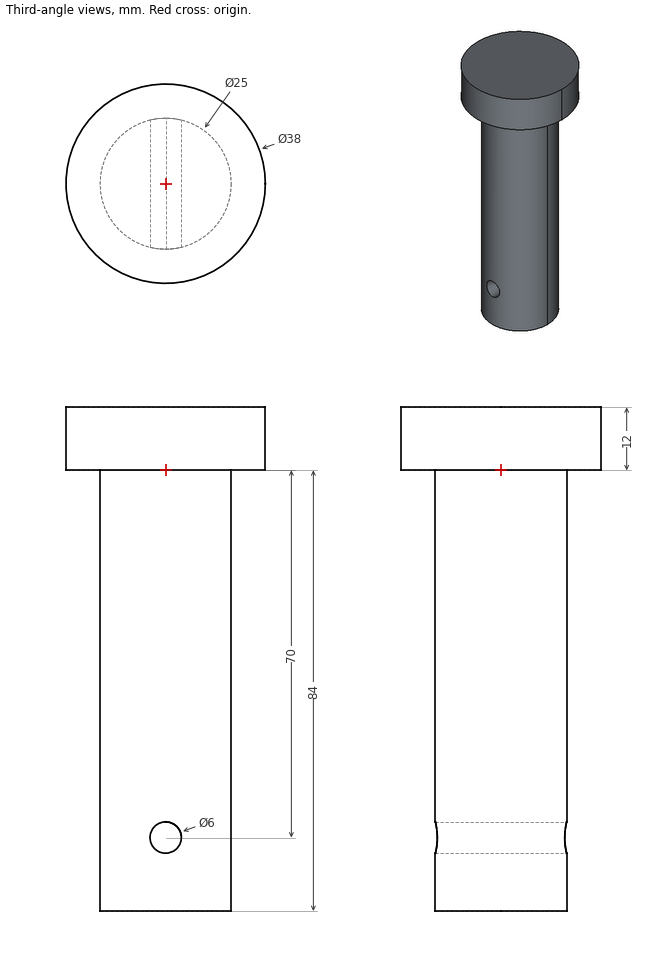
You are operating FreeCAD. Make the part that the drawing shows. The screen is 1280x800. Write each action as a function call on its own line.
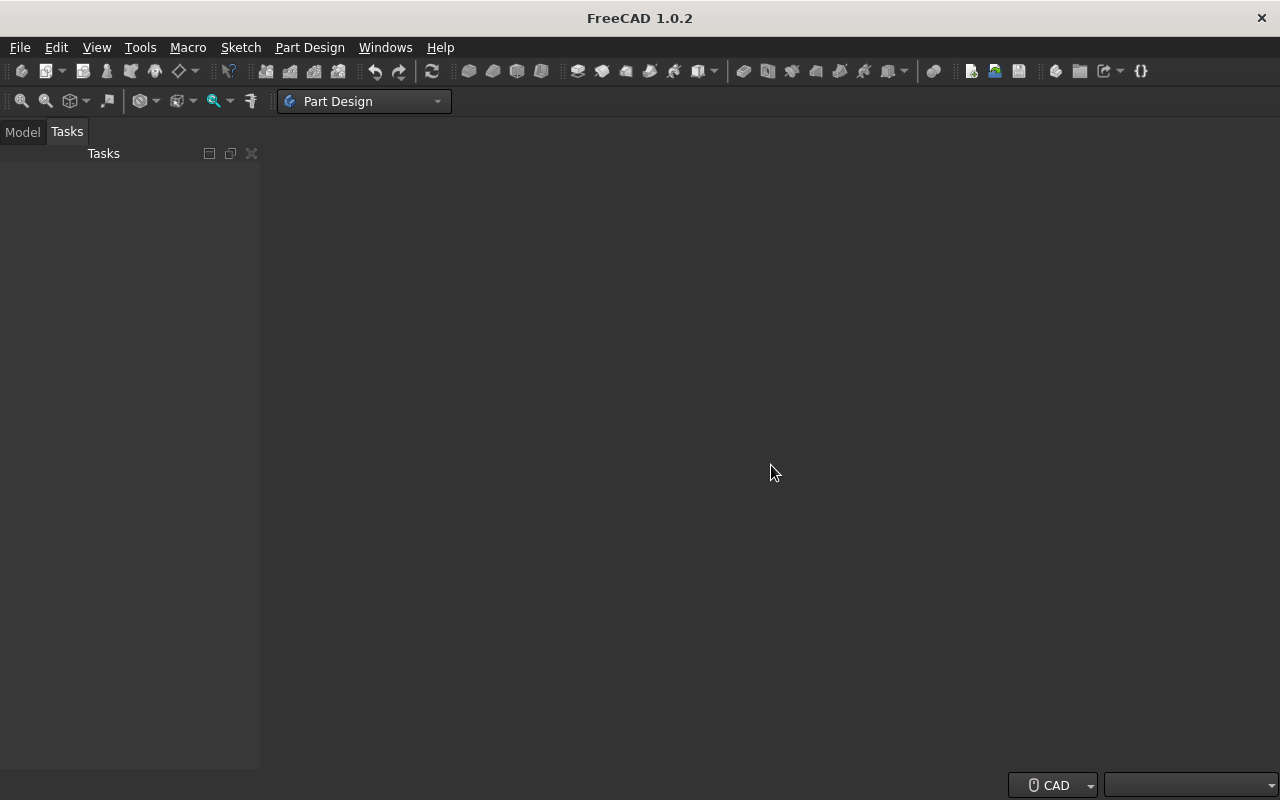
click(972, 72)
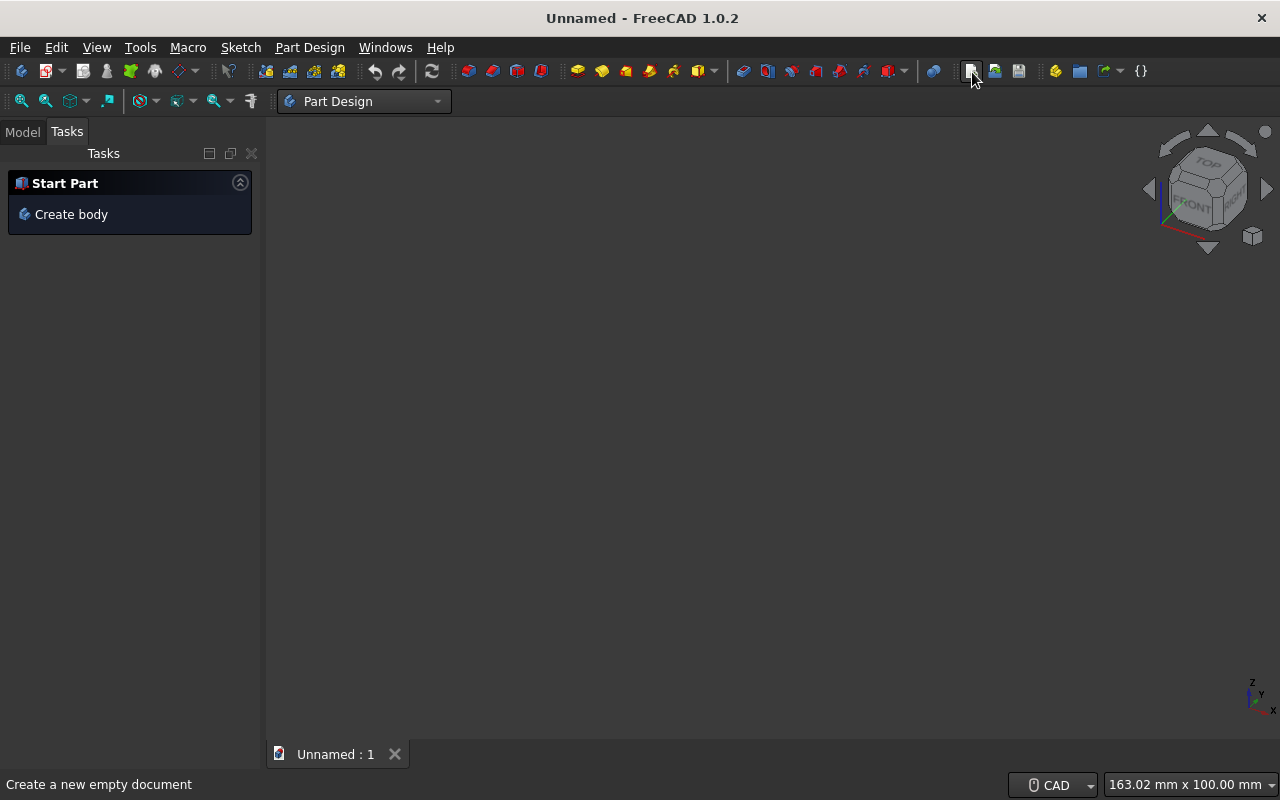
click(46, 72)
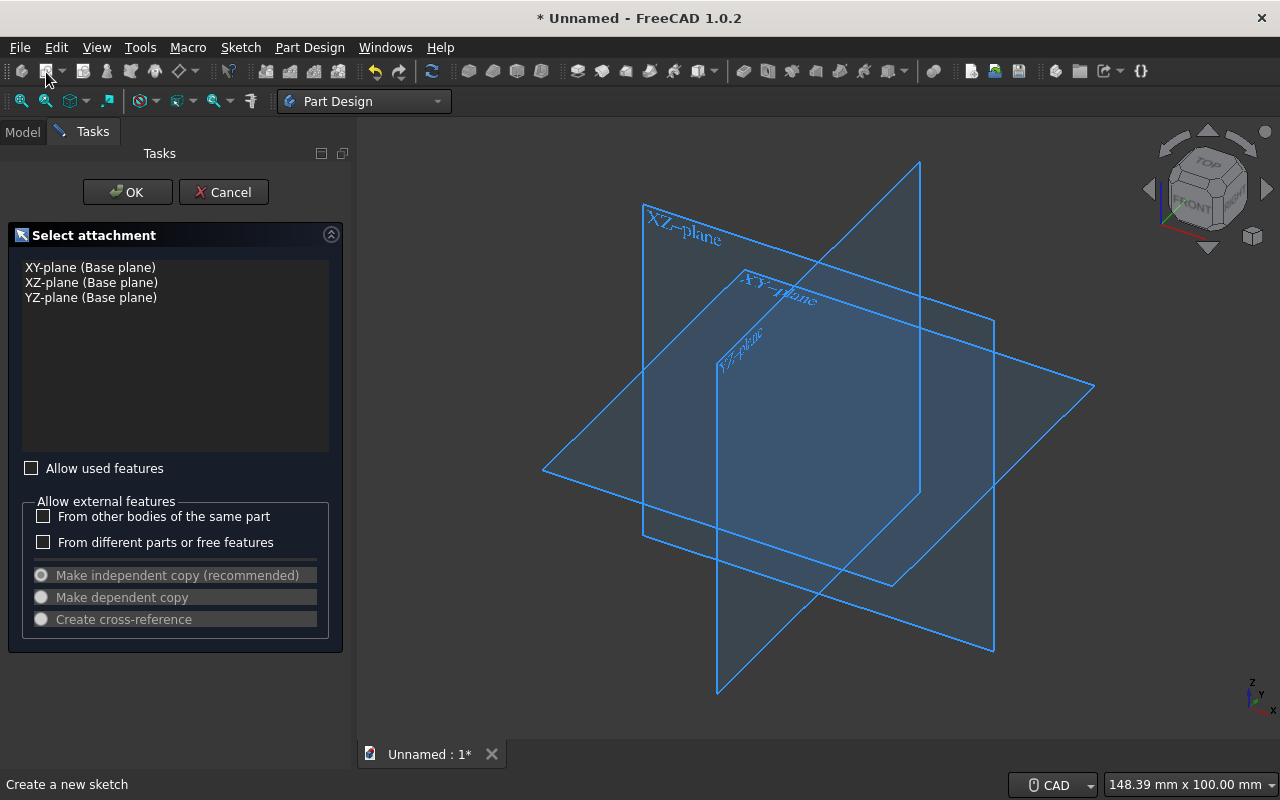
click(82, 268)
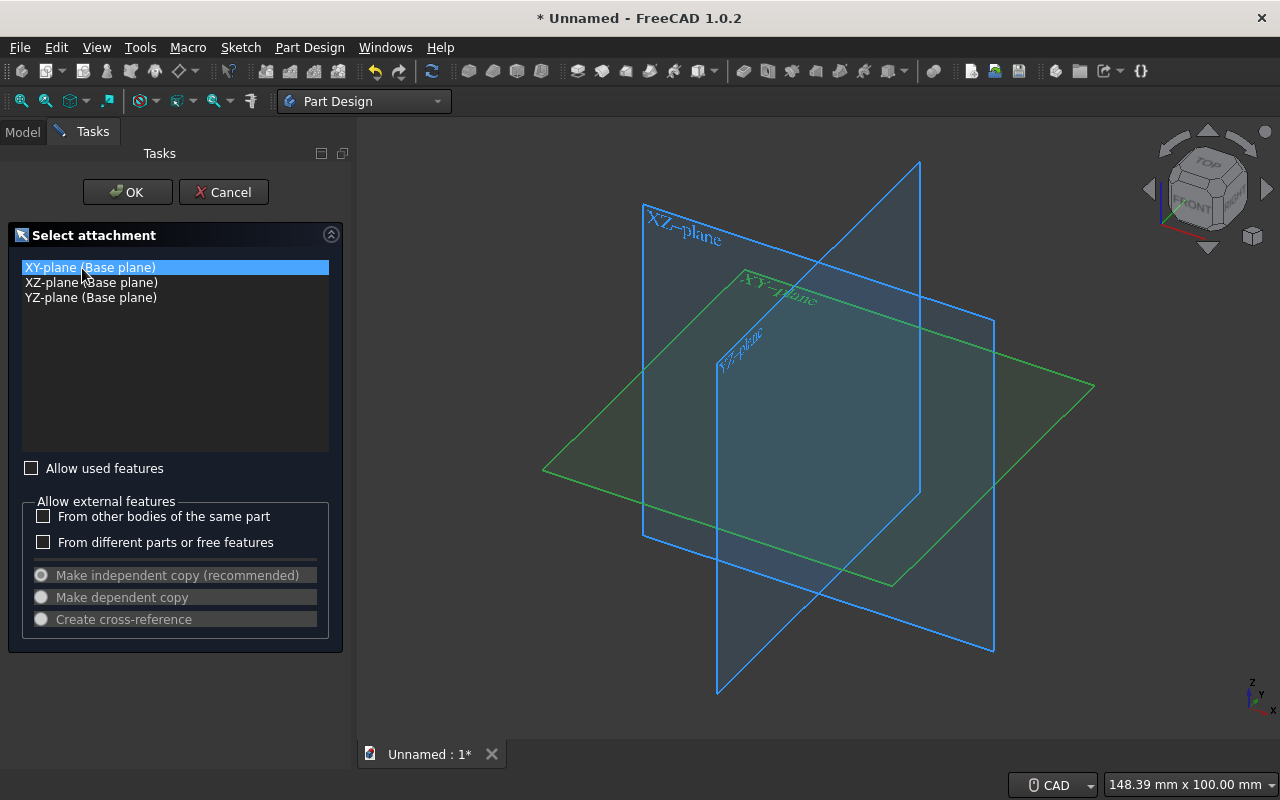
click(128, 192)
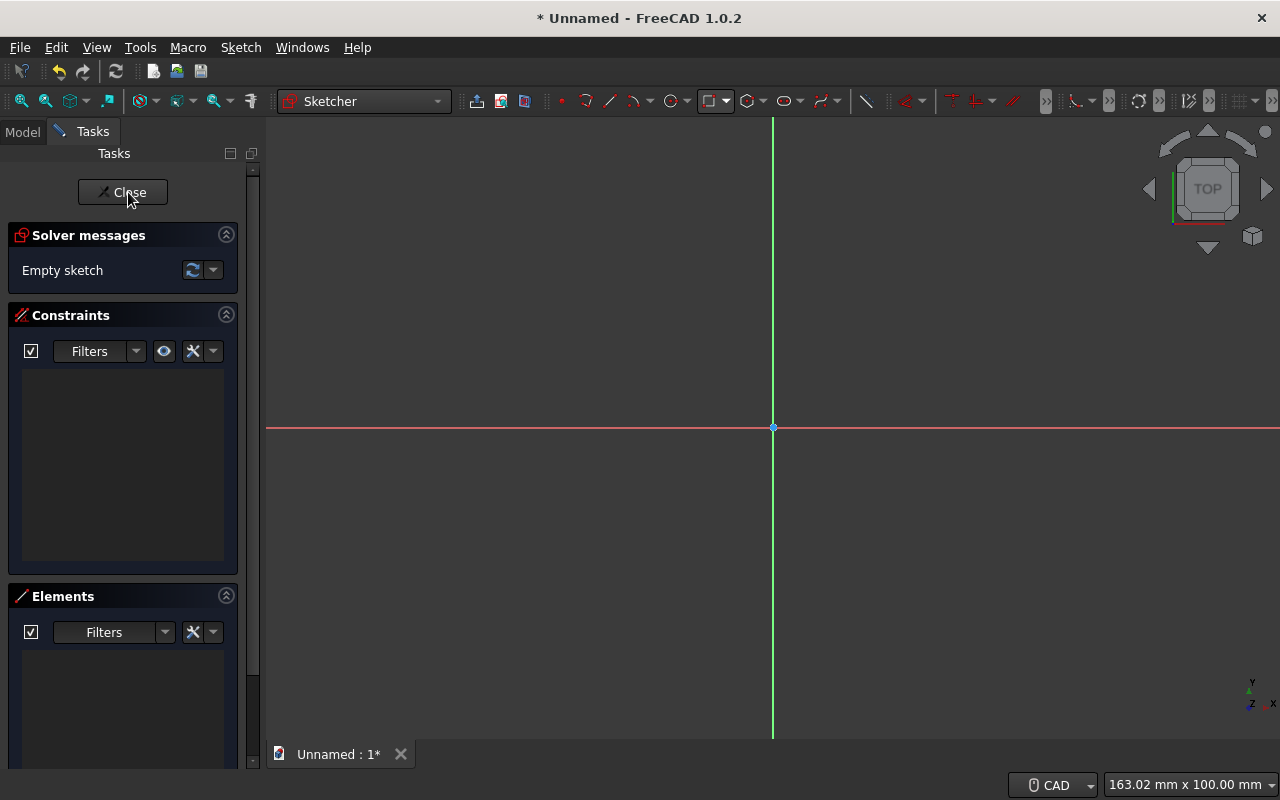
scroll(856, 428, up, 3)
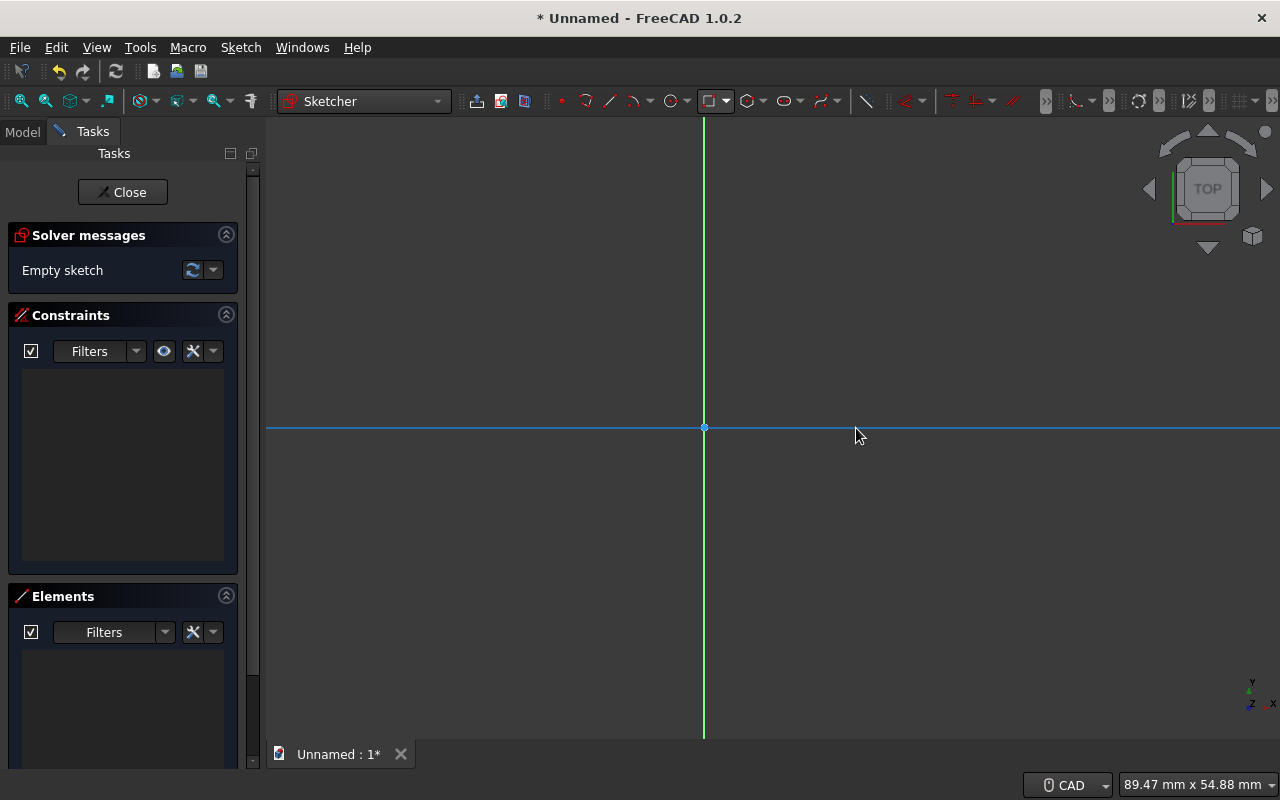
click(672, 102)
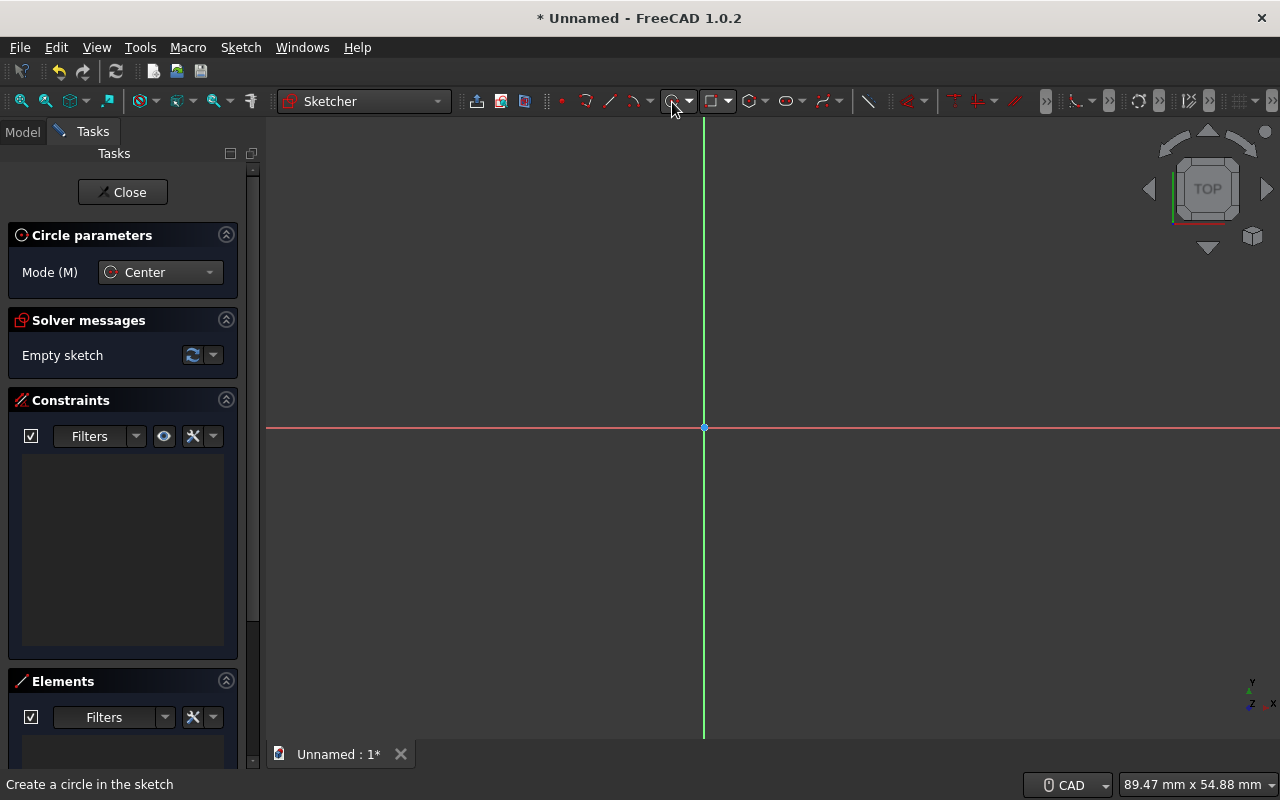
click(704, 428)
click(857, 275)
key(Escape)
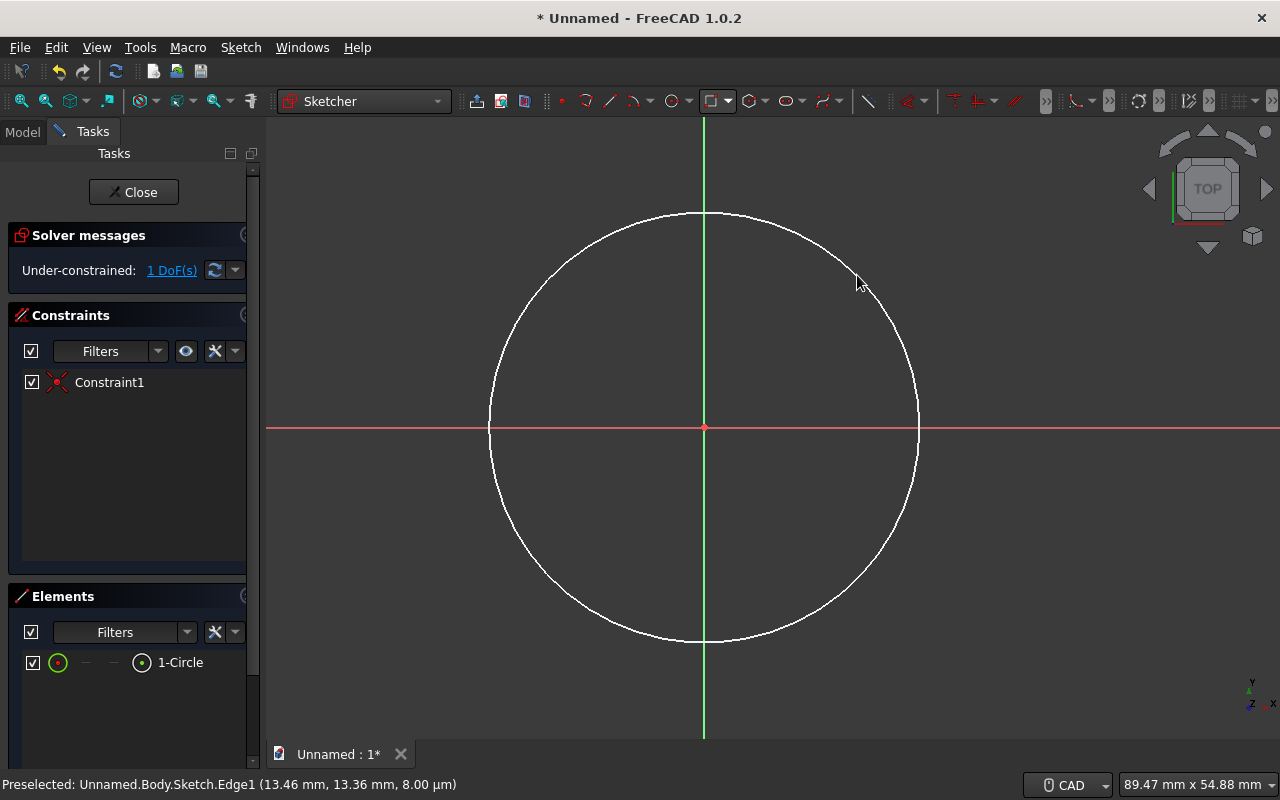
click(908, 102)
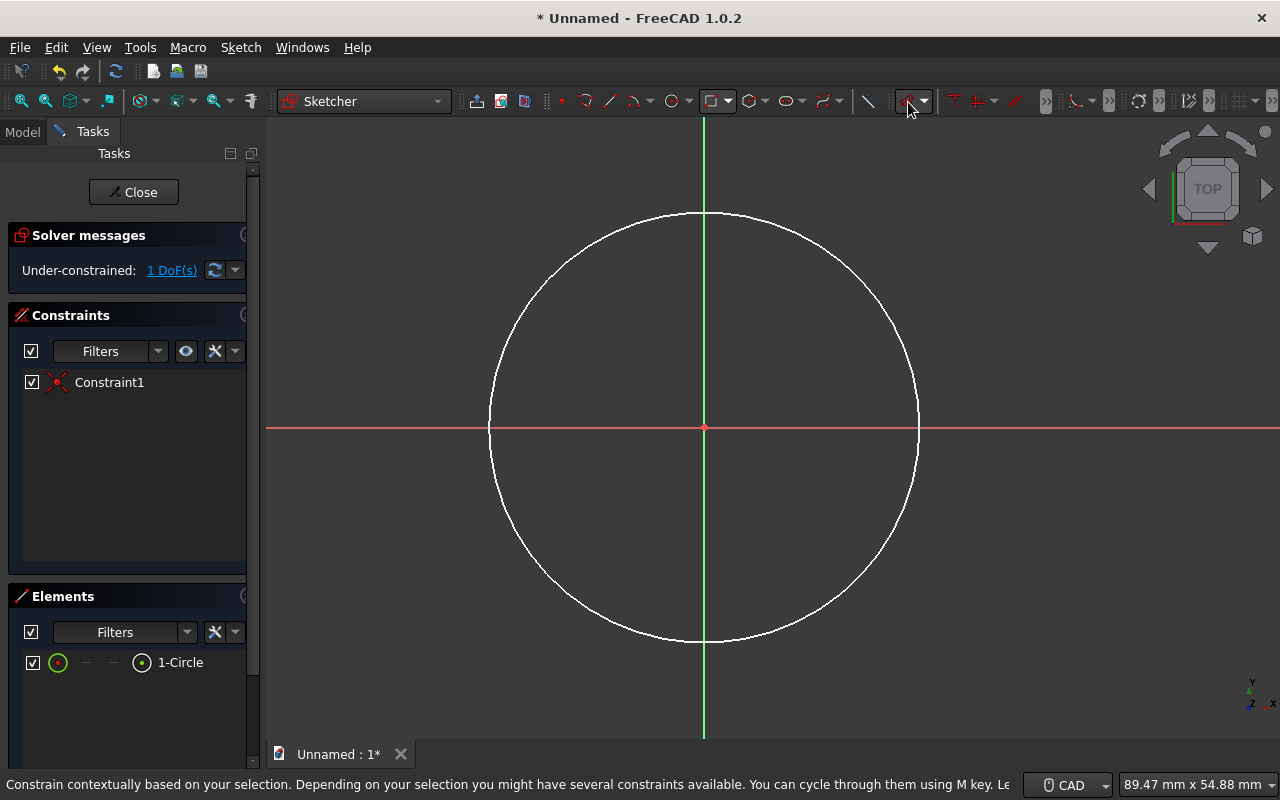
click(856, 275)
click(879, 252)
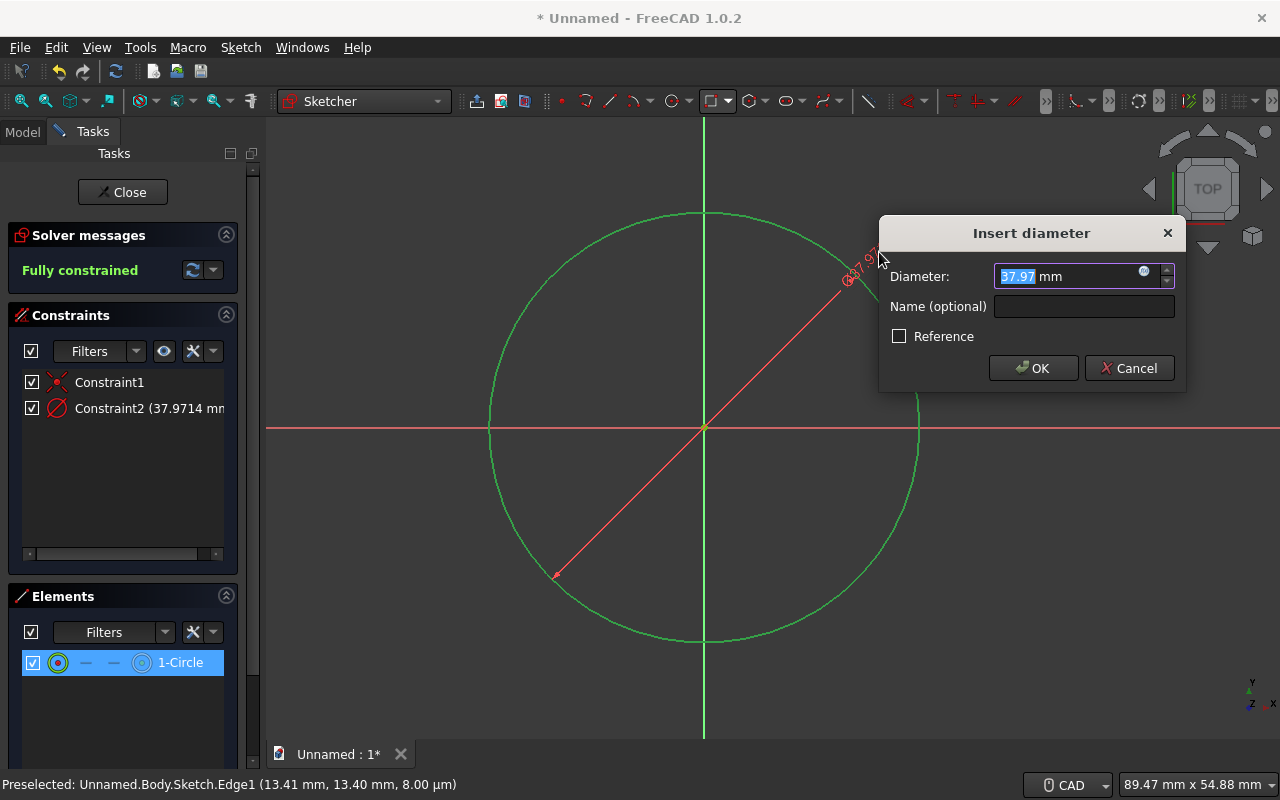
text(38)
key(Return)
key(Escape)